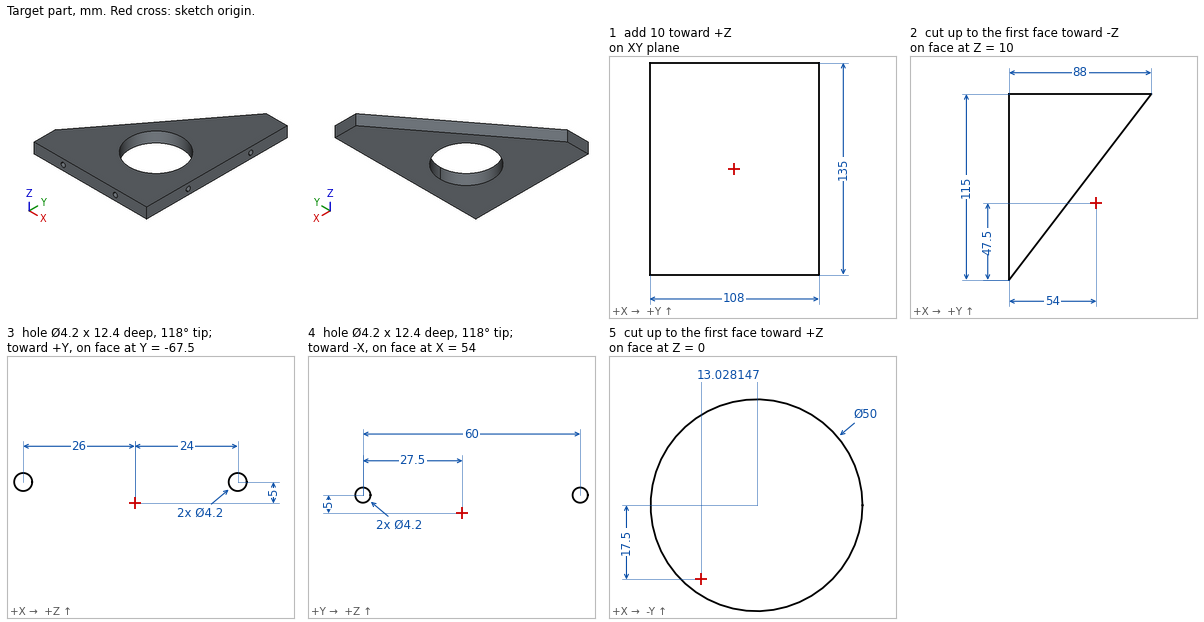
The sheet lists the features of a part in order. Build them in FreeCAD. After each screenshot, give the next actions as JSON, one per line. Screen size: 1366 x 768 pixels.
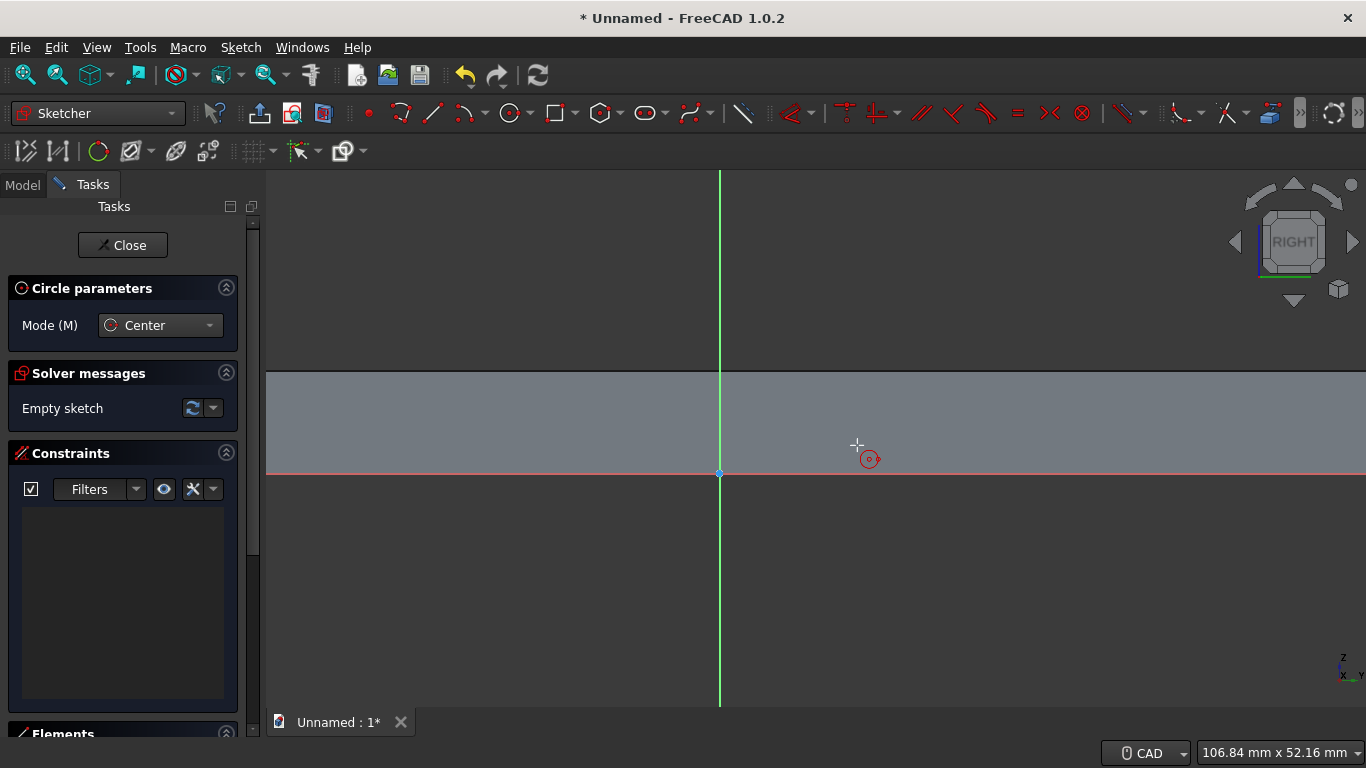
{"action": "left_click", "coordinate": [437, 422]}
{"action": "mouse_move", "coordinate": [452, 407]}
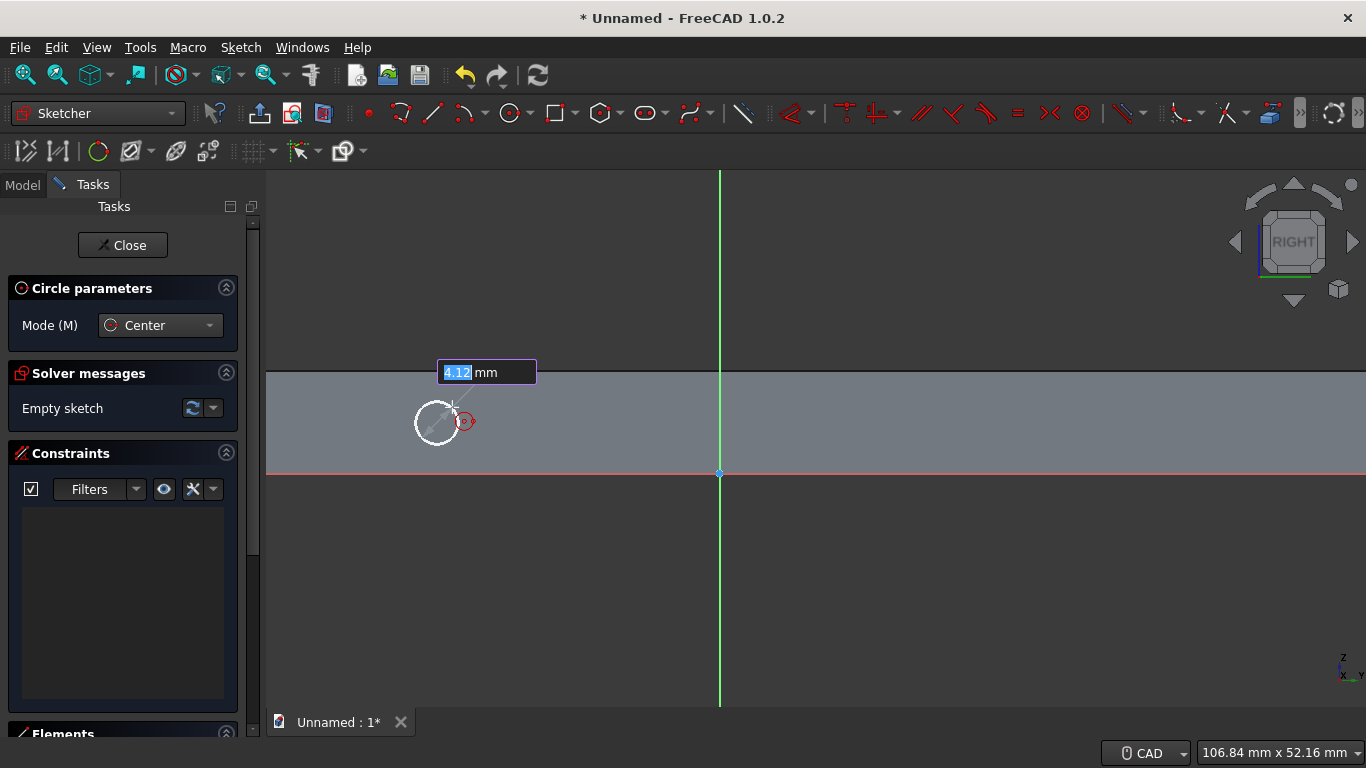
{"action": "type", "text": "4.2"}
{"action": "key", "text": "Return"}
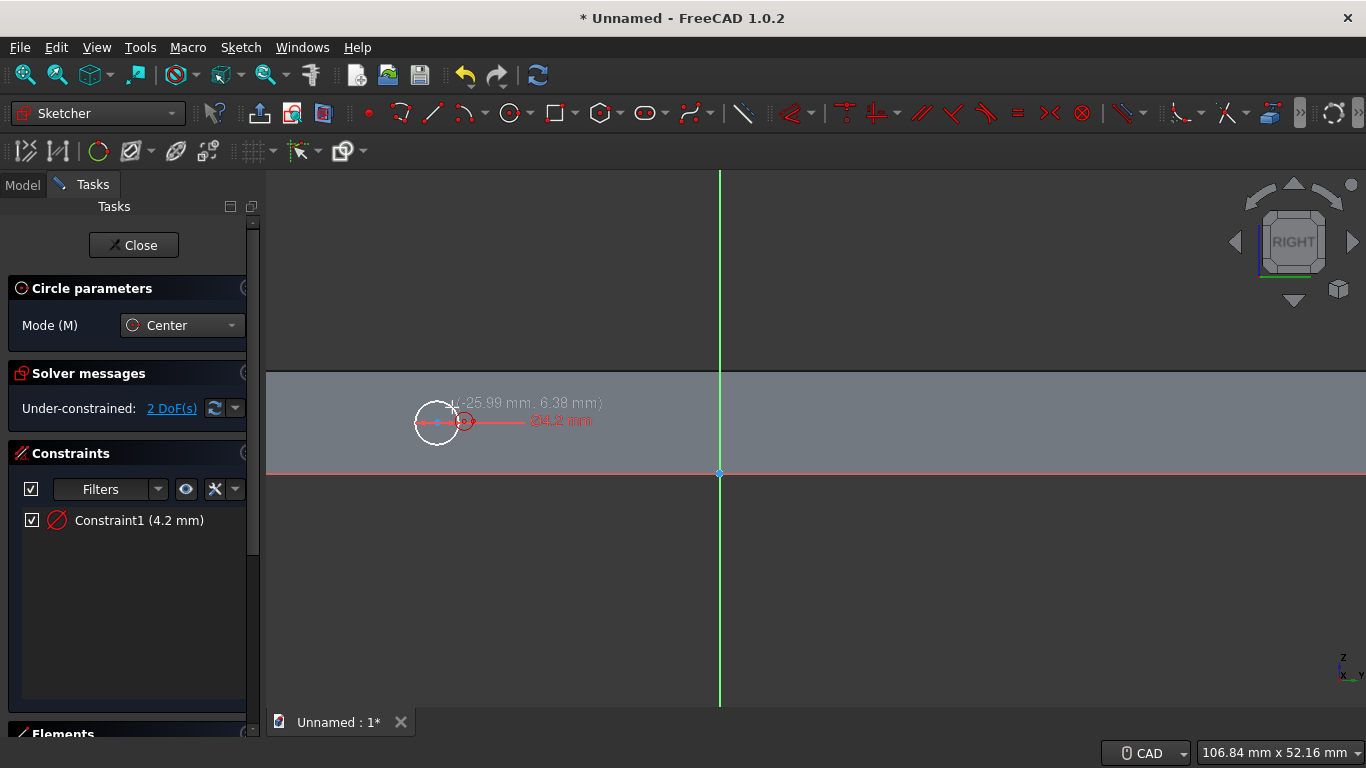
{"action": "left_click", "coordinate": [1054, 422]}
{"action": "mouse_move", "coordinate": [1070, 407]}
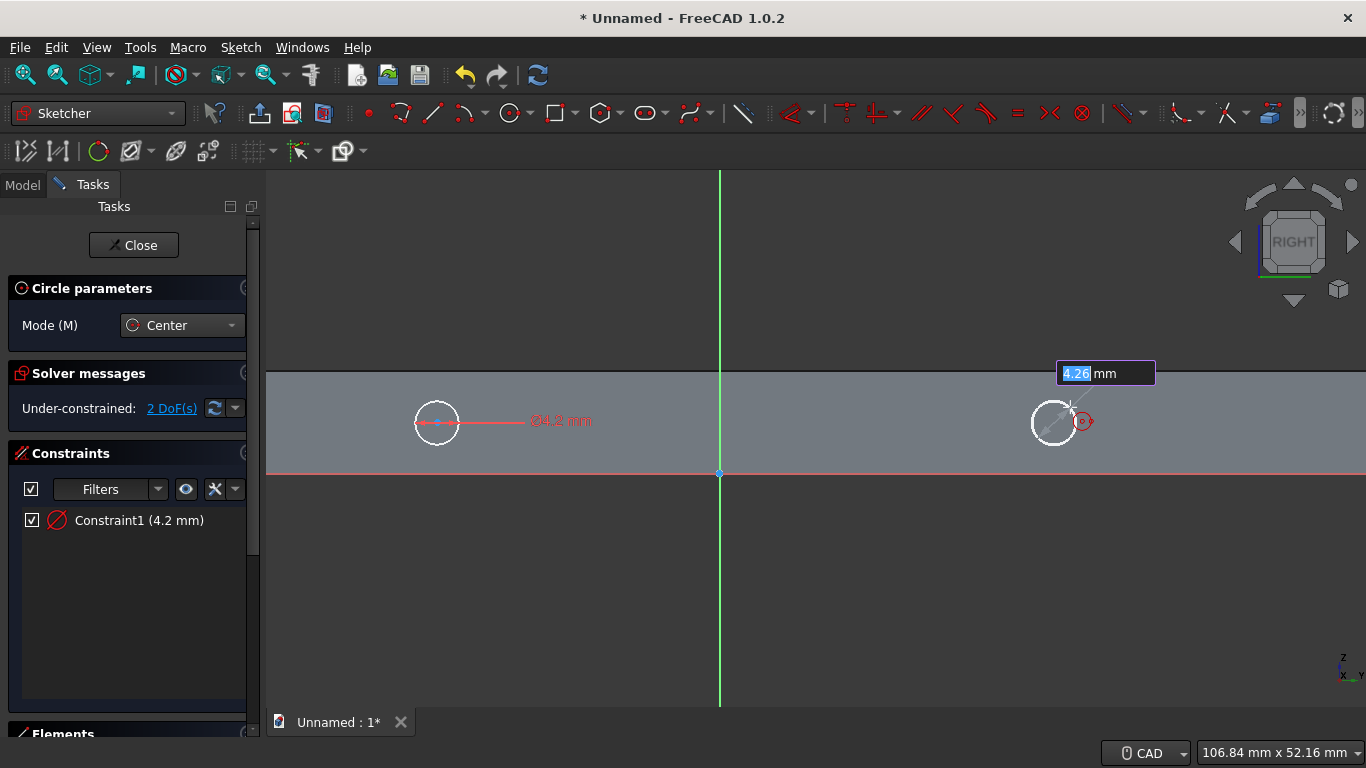
{"action": "type", "text": "4.2"}
{"action": "key", "text": "Return"}
{"action": "key", "text": "Escape"}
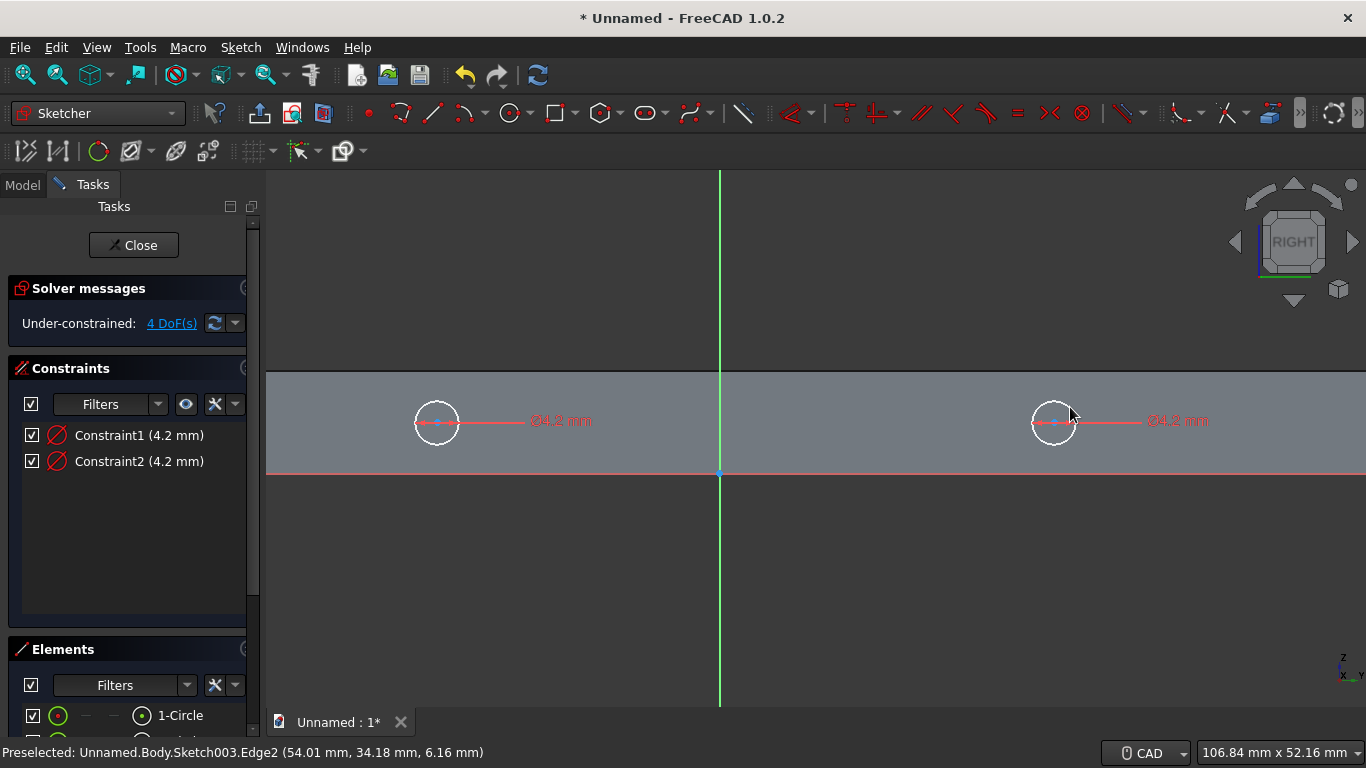
{"action": "left_click", "coordinate": [437, 423]}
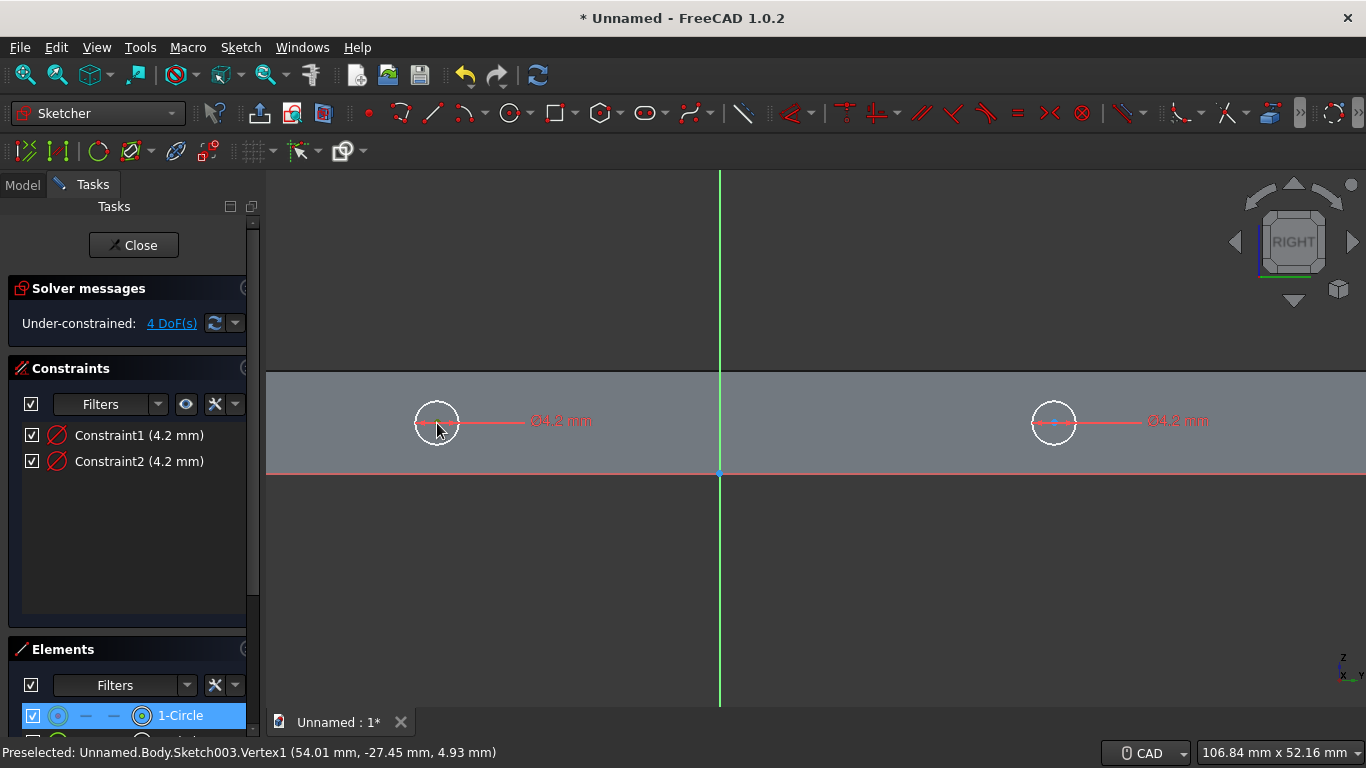
{"action": "left_click", "coordinate": [1054, 423]}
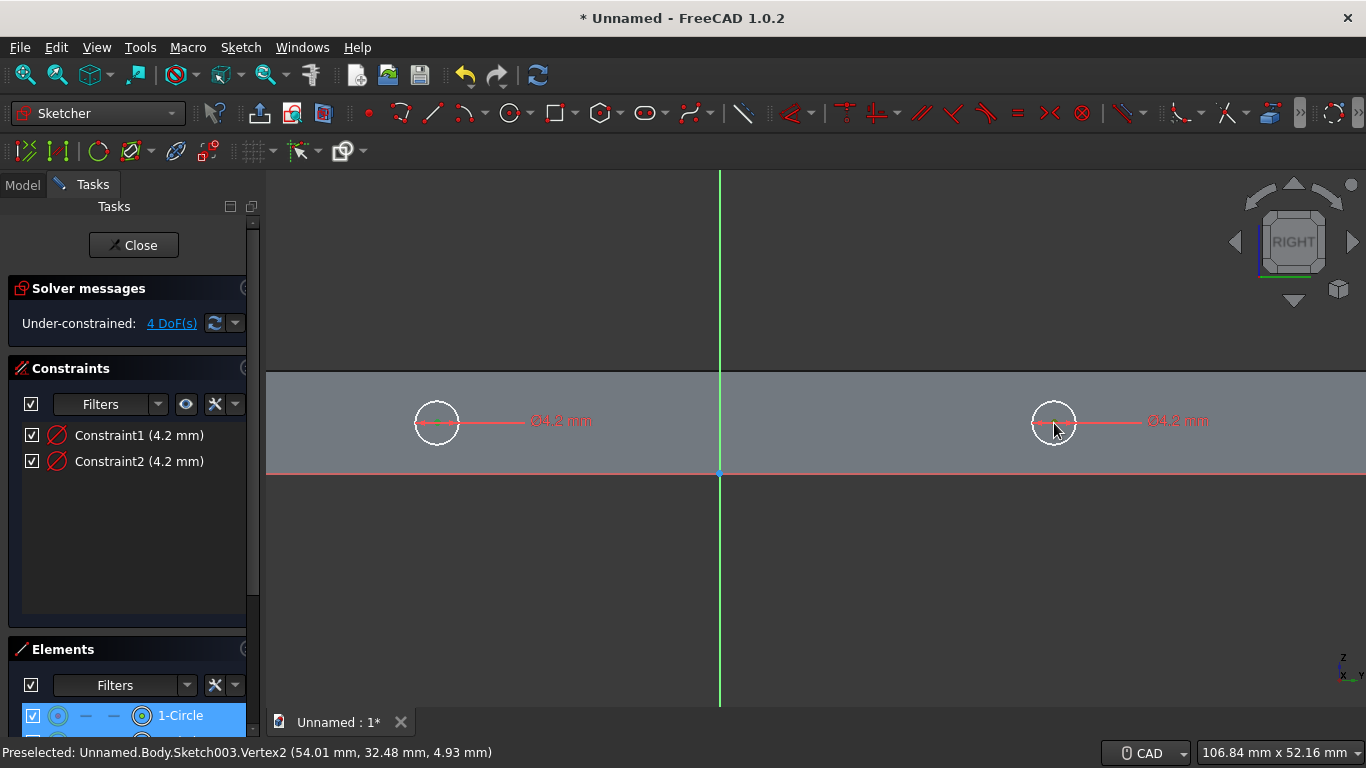
{"action": "left_click", "coordinate": [900, 114]}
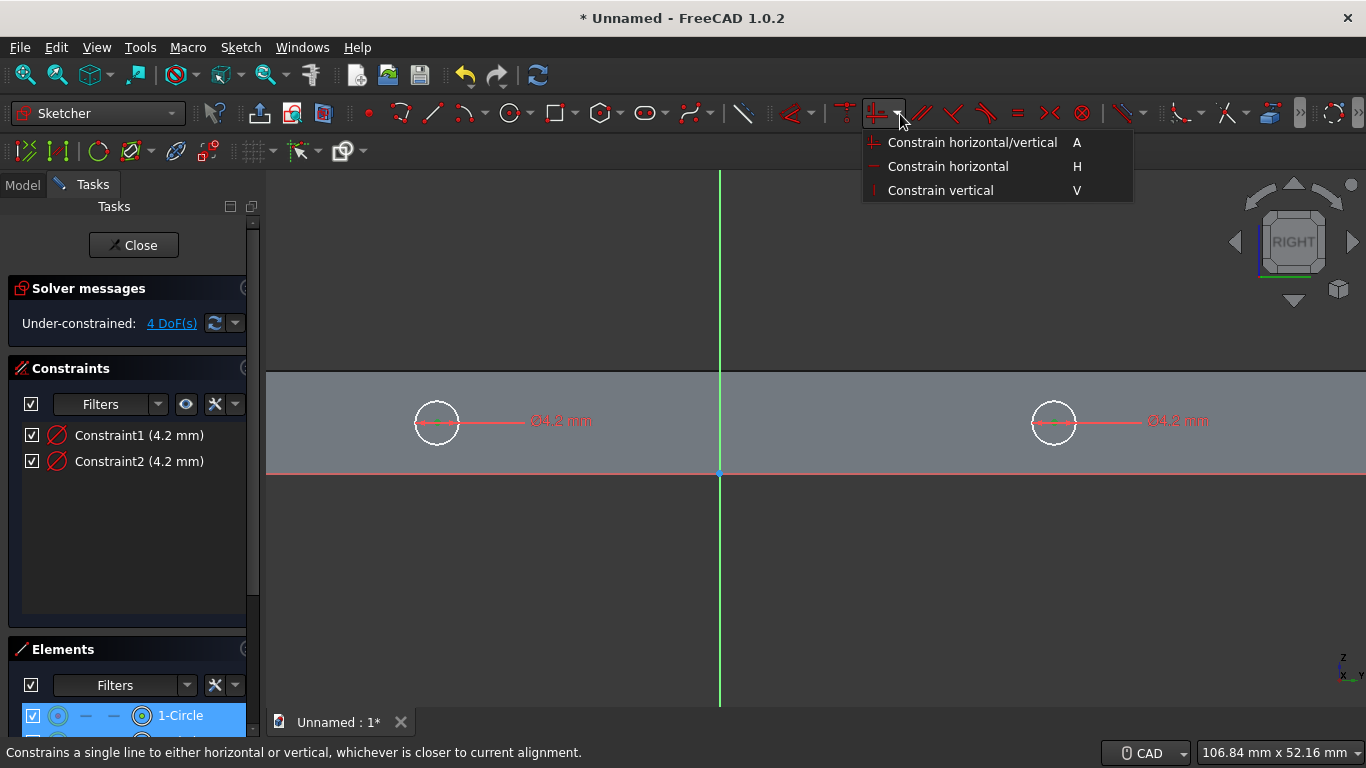
{"action": "left_click", "coordinate": [998, 166]}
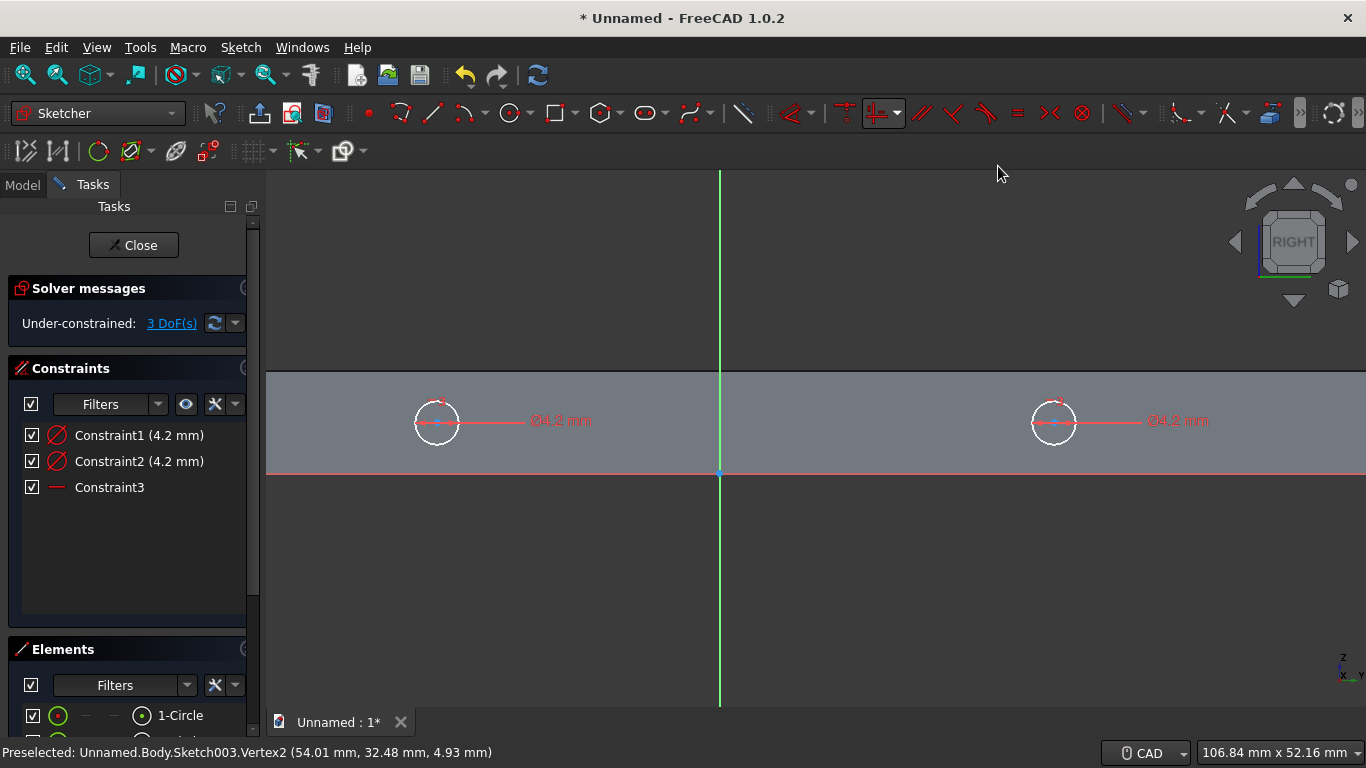
{"action": "key", "text": "d"}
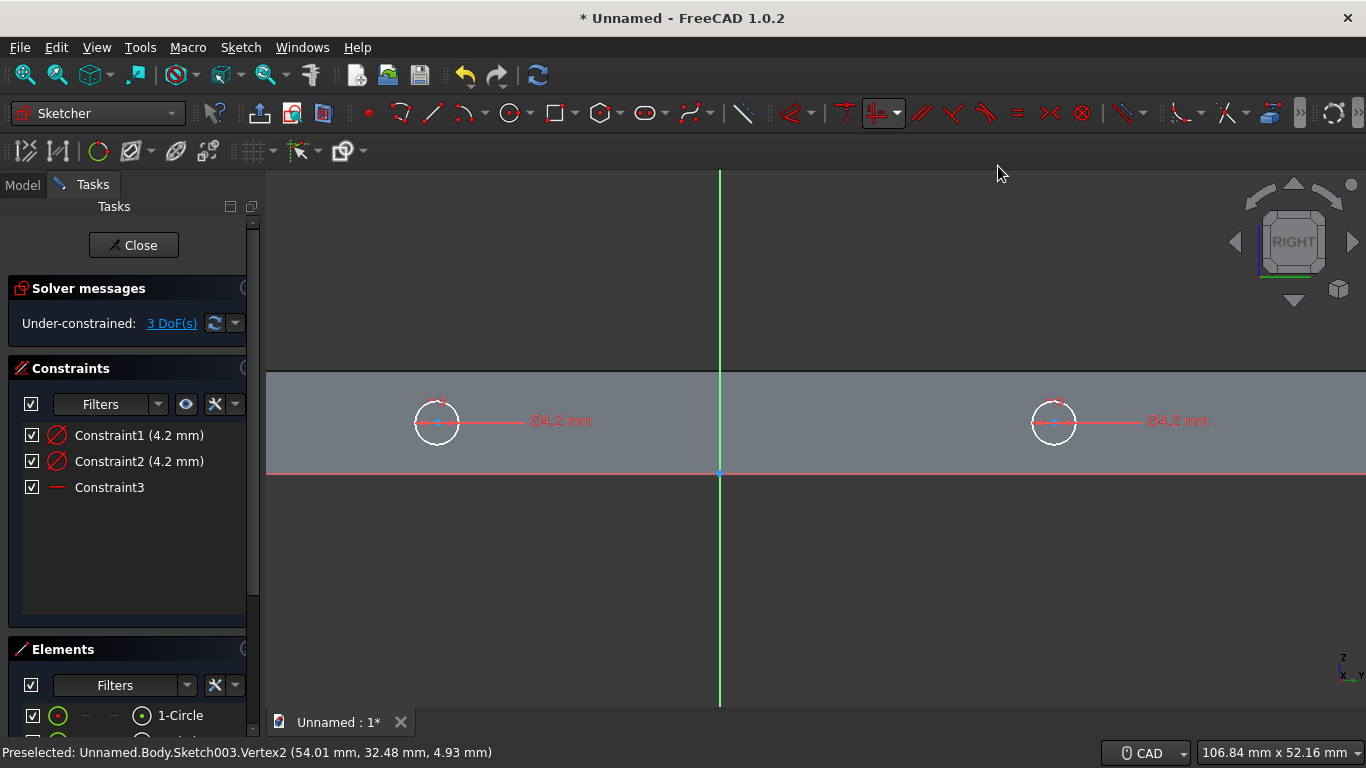
{"action": "left_click", "coordinate": [437, 423]}
{"action": "left_click", "coordinate": [403, 448]}